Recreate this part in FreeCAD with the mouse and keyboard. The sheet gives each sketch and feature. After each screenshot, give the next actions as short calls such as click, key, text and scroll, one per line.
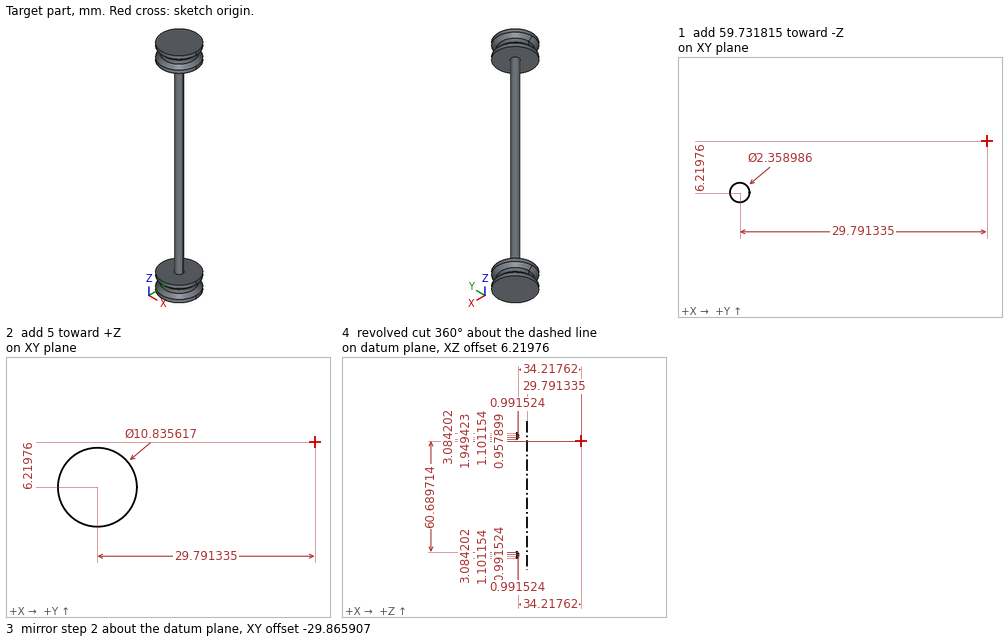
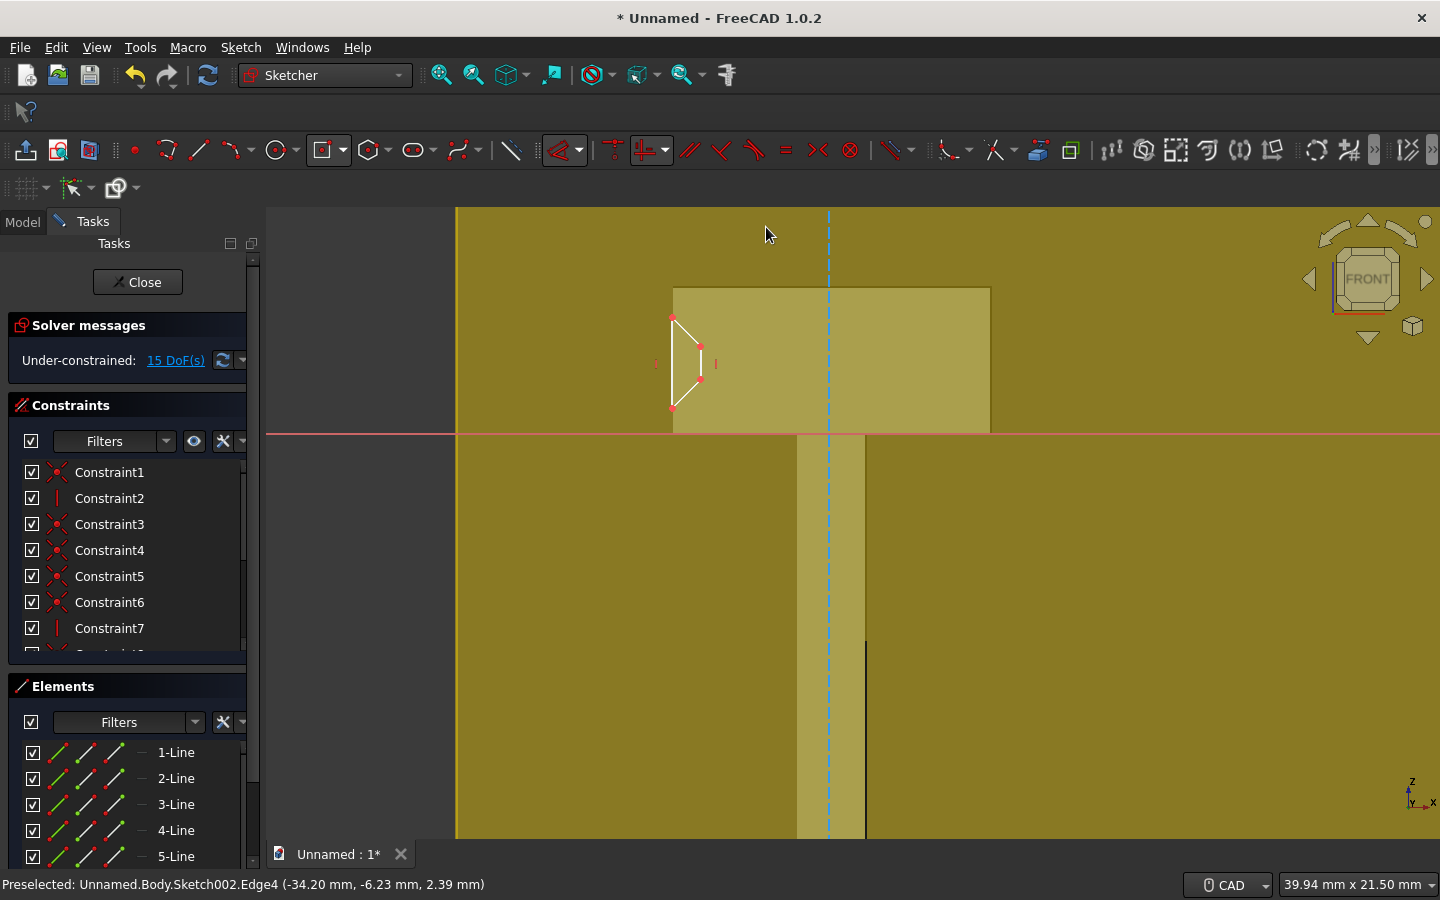
click(672, 381)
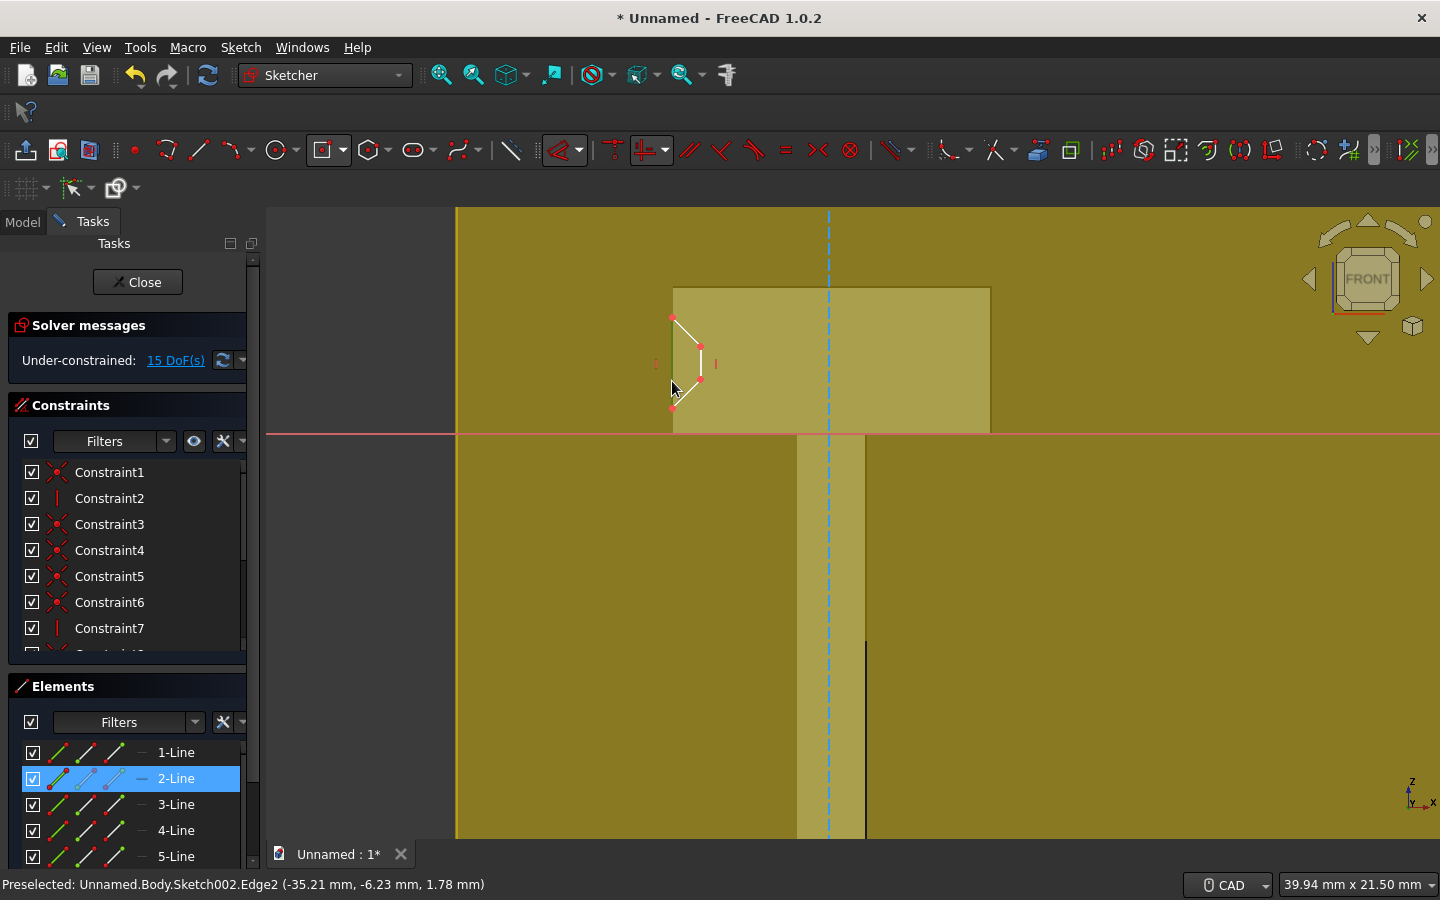
click(582, 150)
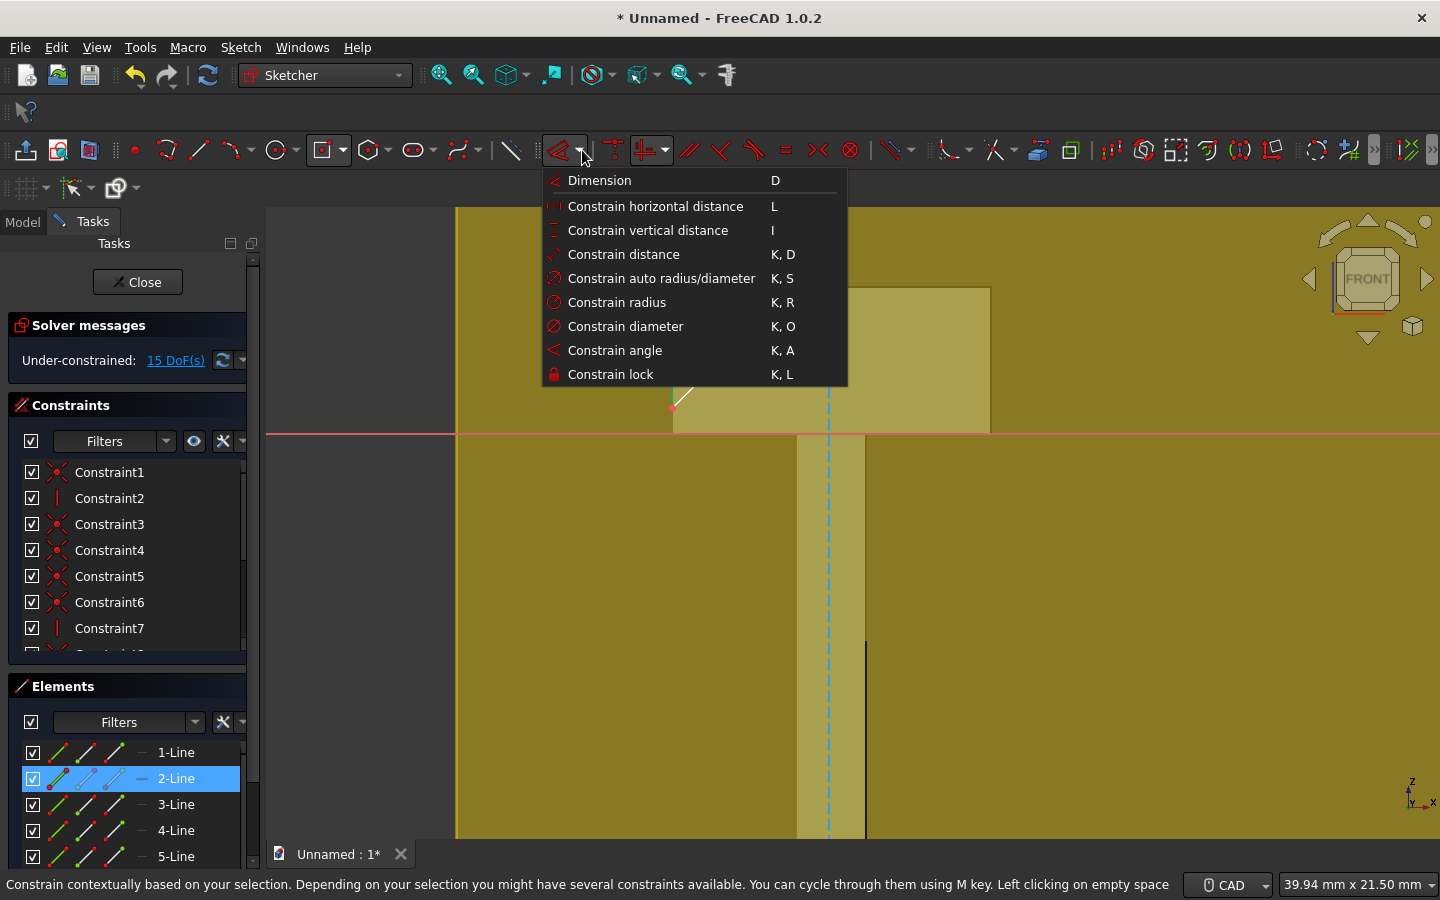
click(695, 230)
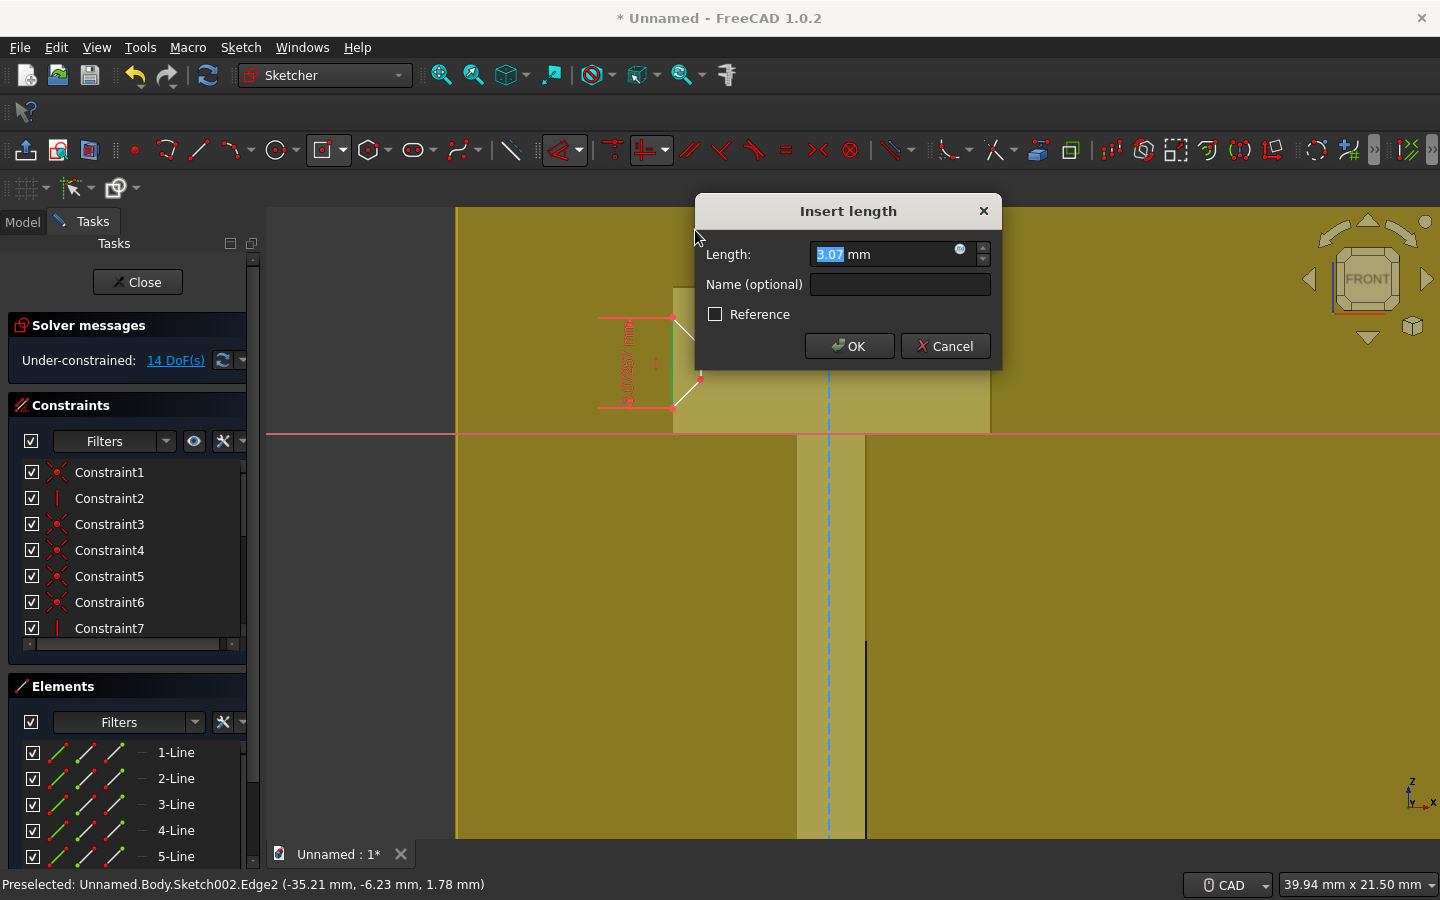
text(3.084202)
key(Return)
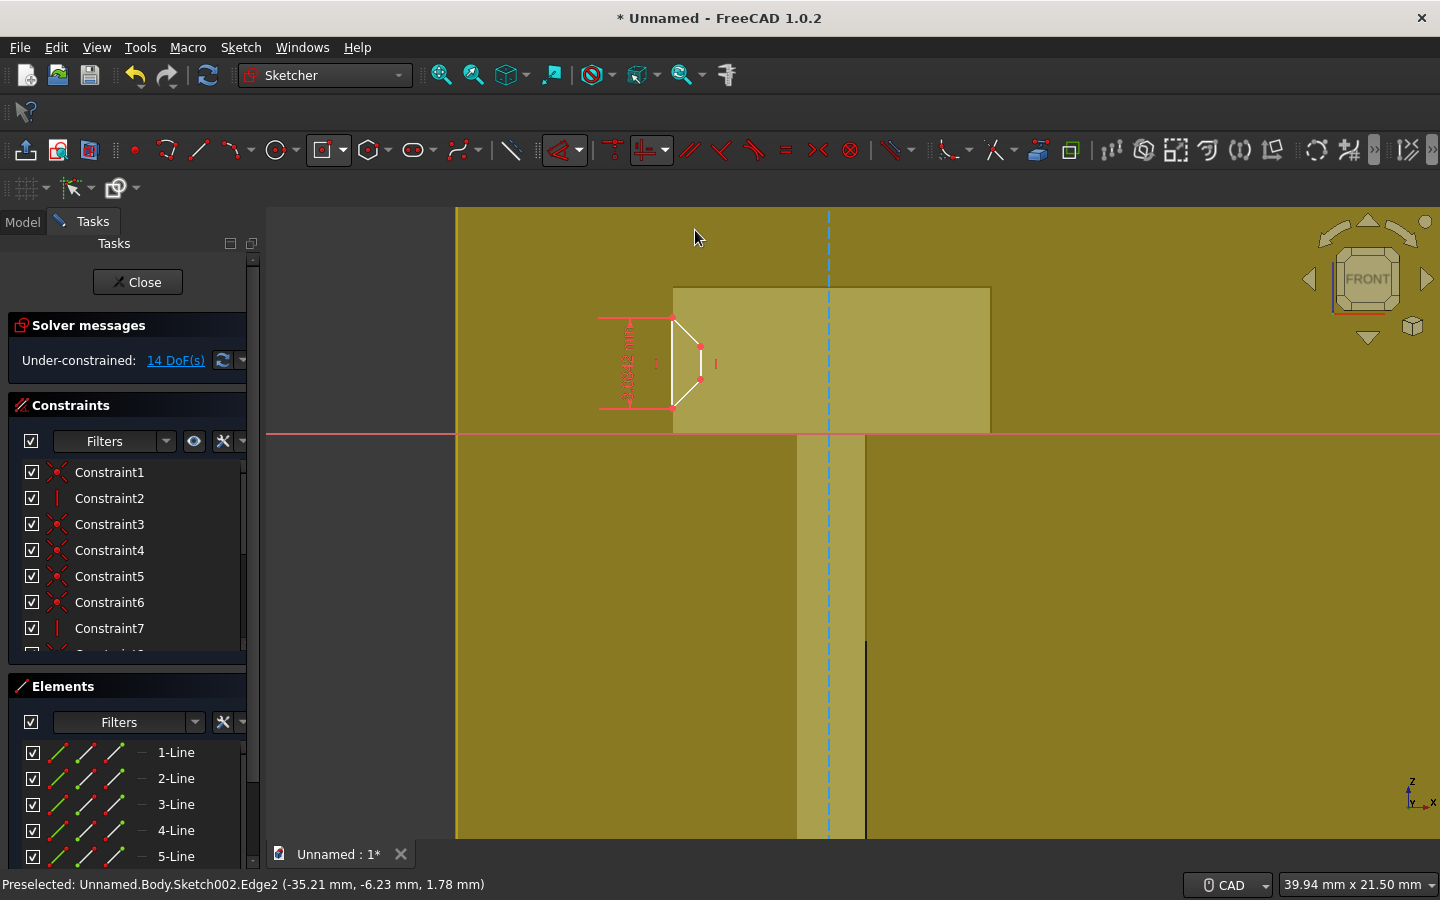
scroll(701, 357, up, 2)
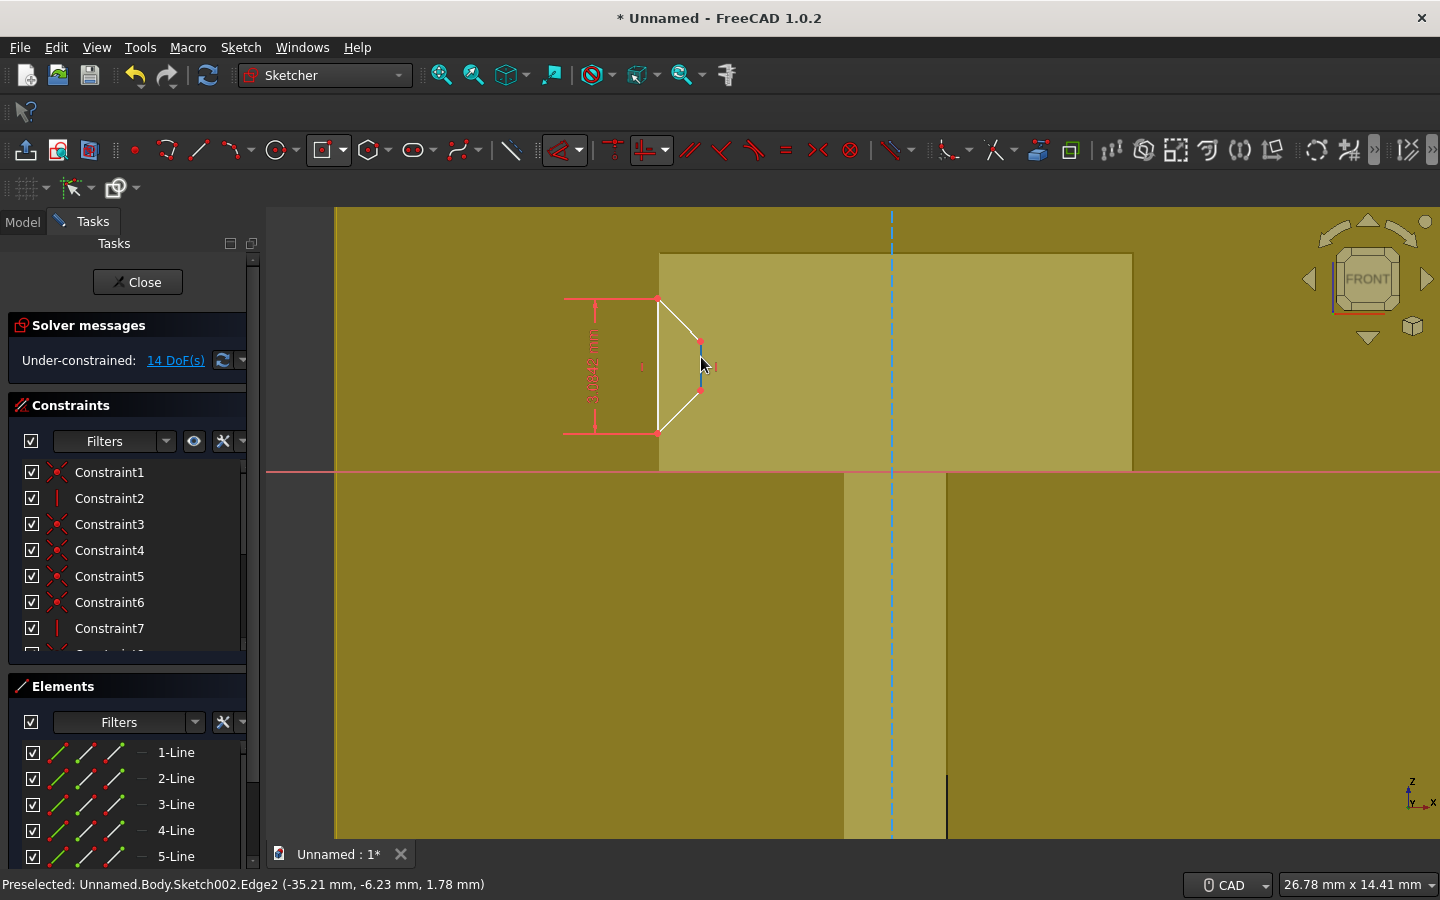
click(701, 356)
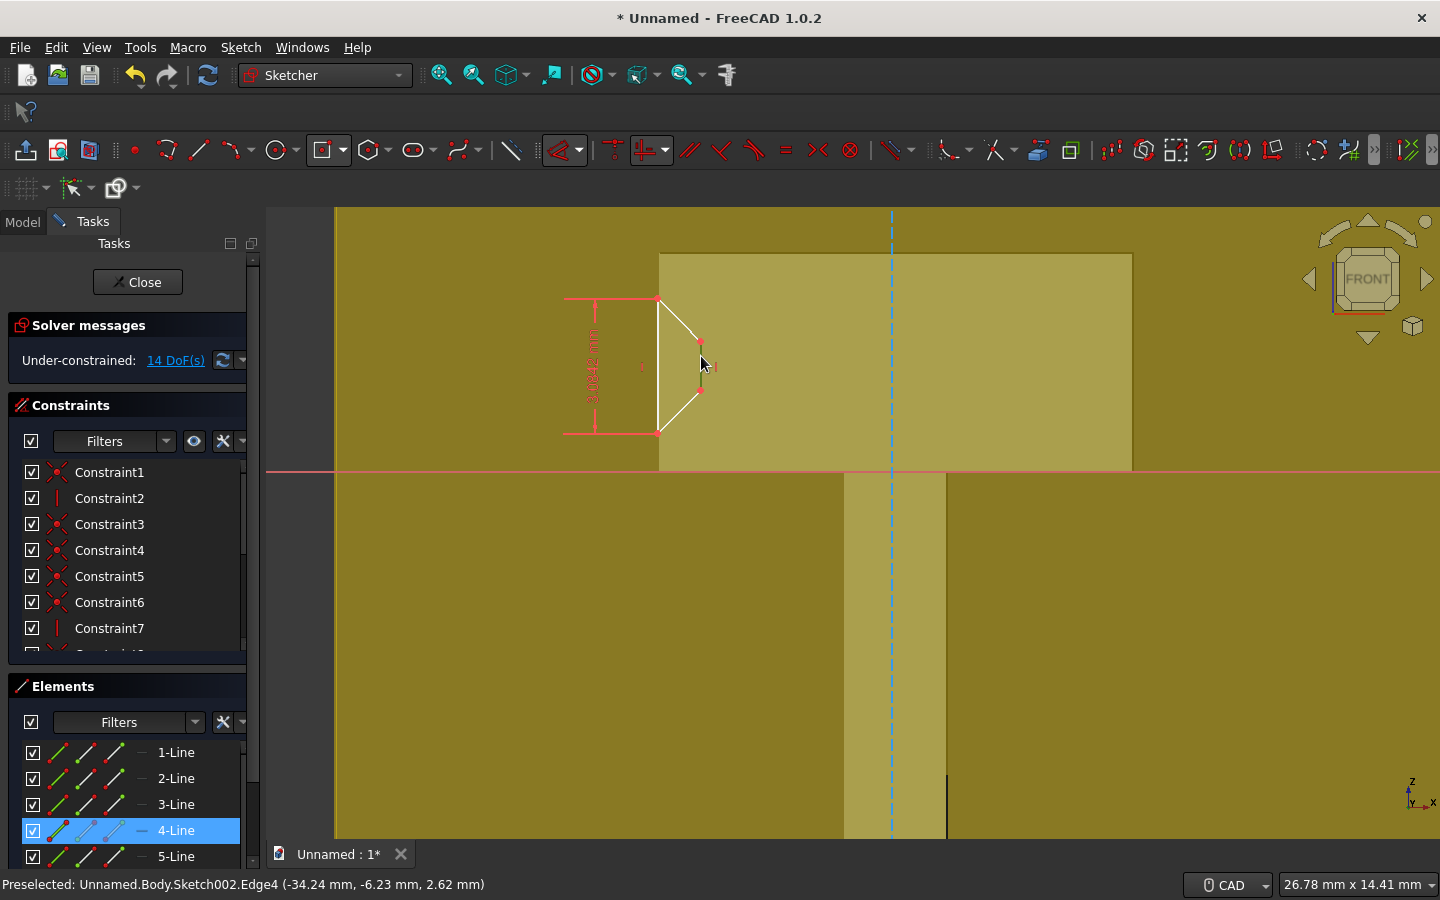
key(i)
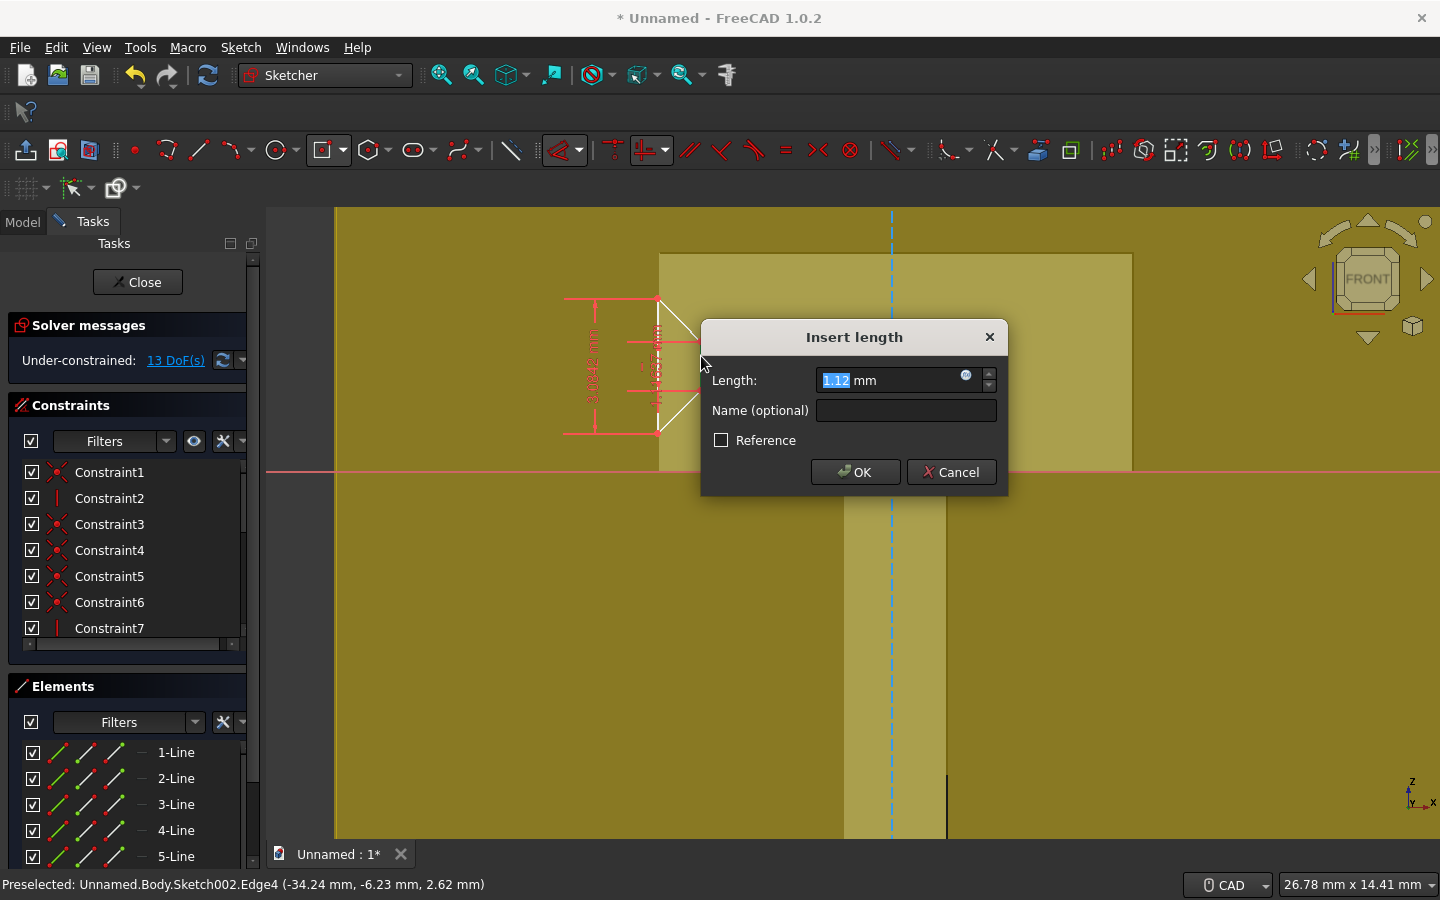
text(1.101154)
key(Return)